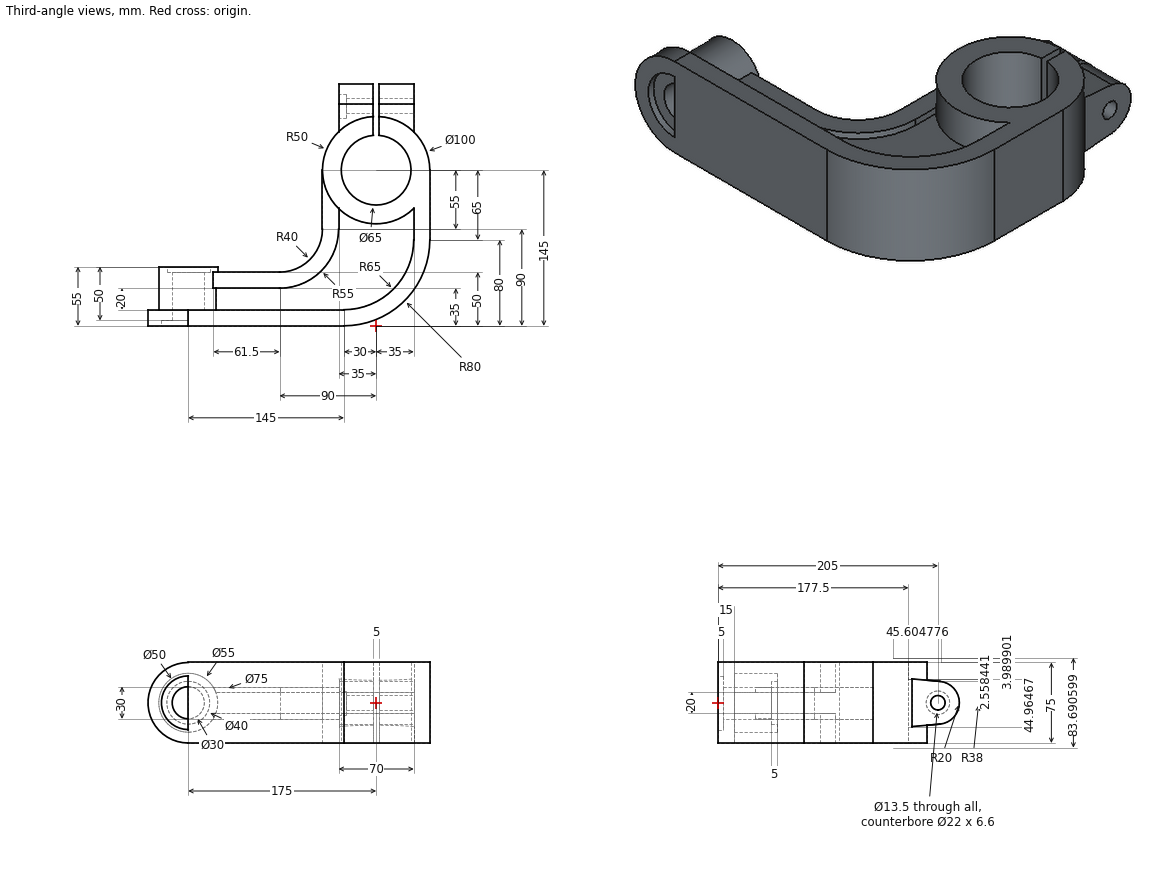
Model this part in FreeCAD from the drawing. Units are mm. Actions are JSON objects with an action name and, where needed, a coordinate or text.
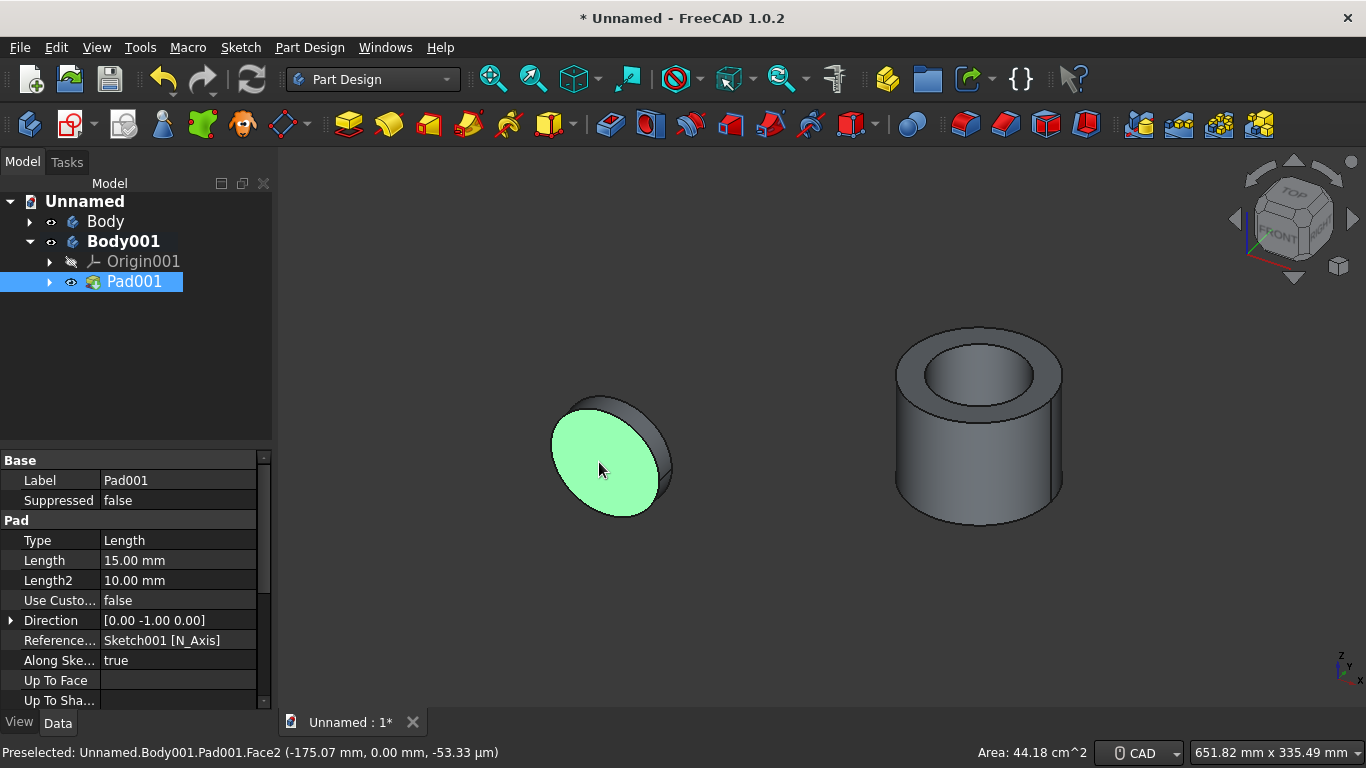
{"action": "left_click", "coordinate": [70, 124]}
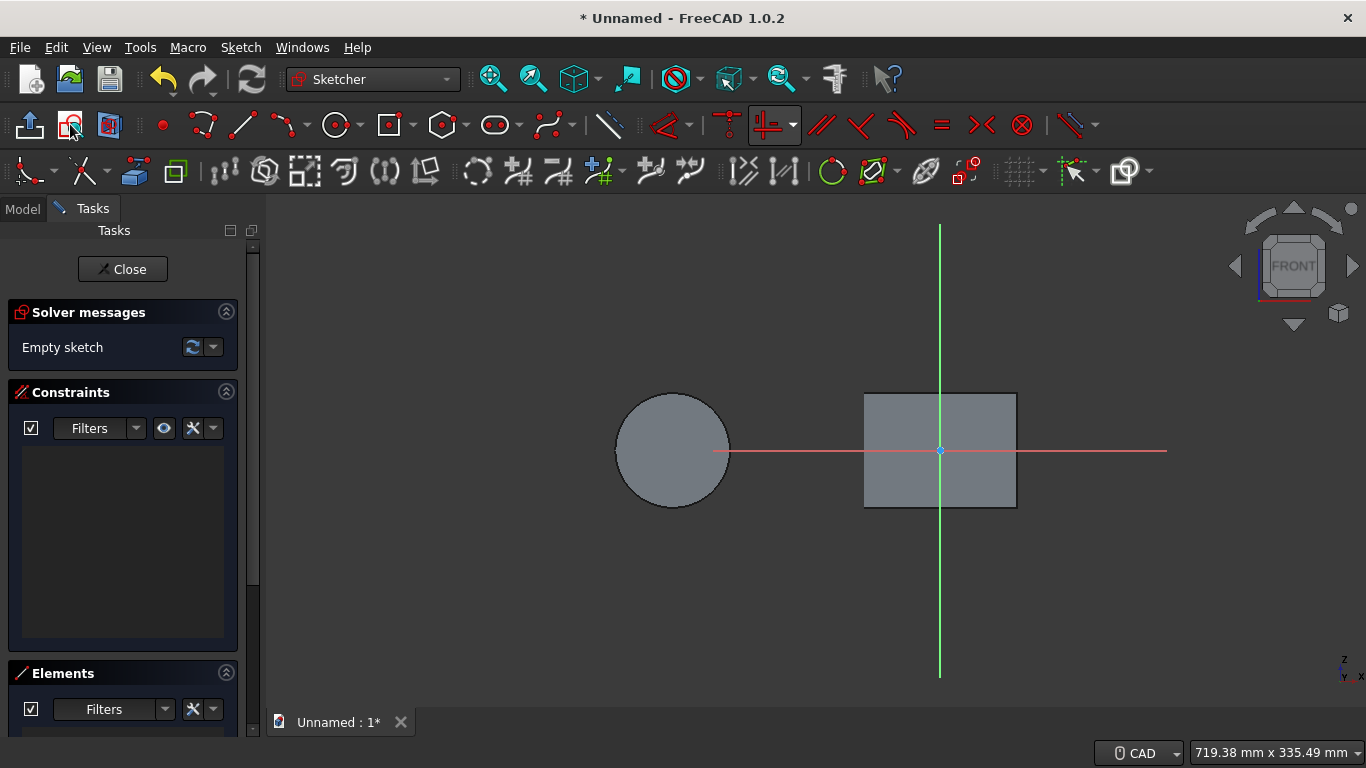
{"action": "scroll", "coordinate": [648, 450], "scroll_direction": "up", "scroll_amount": 7}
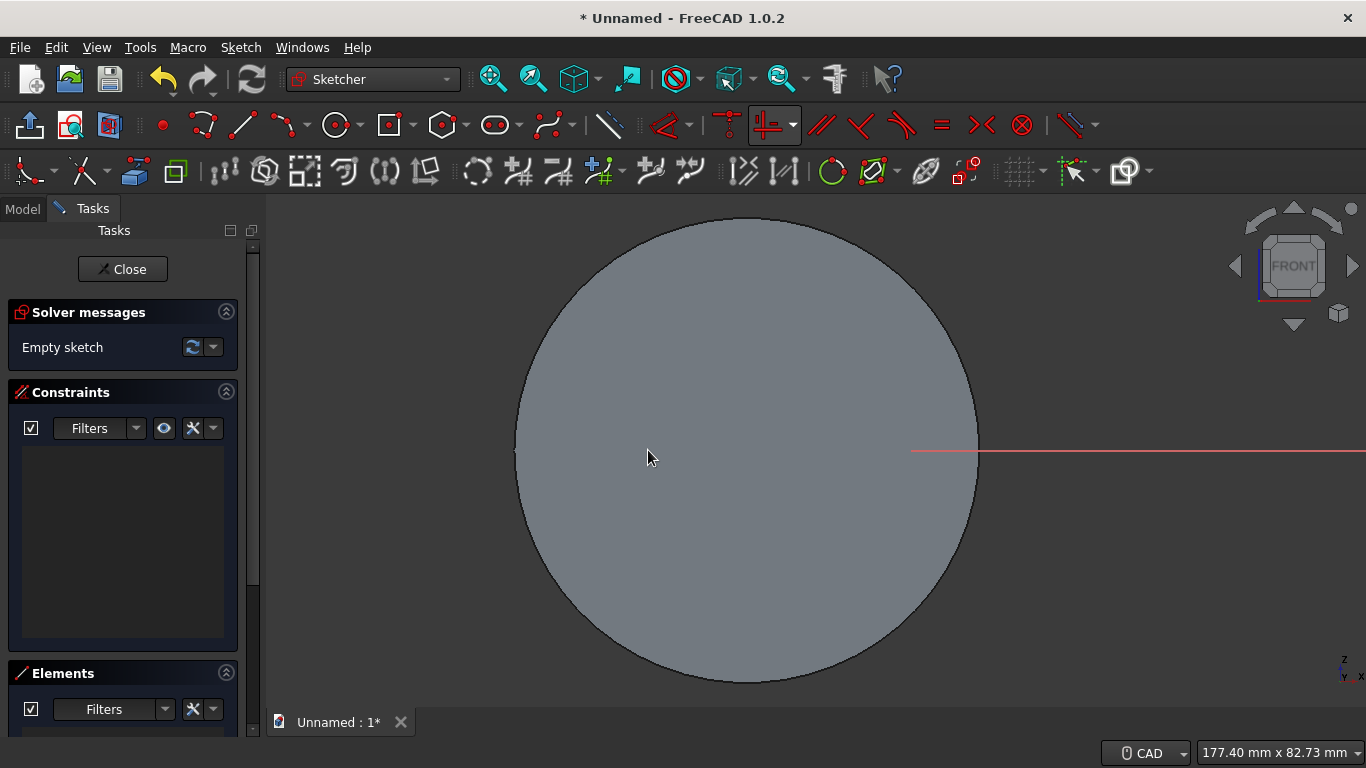
{"action": "key", "text": "g c"}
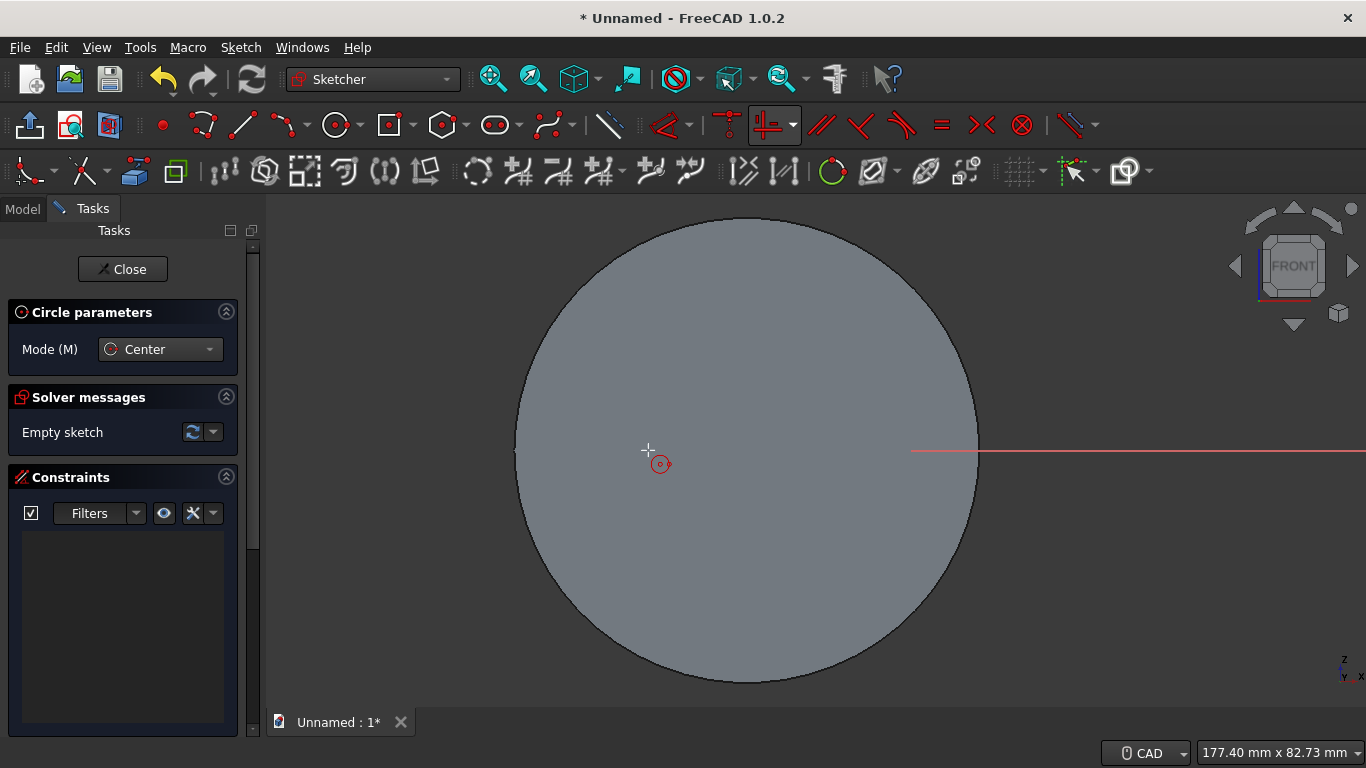
{"action": "left_click", "coordinate": [747, 450]}
{"action": "left_click", "coordinate": [867, 330]}
{"action": "key", "text": "Escape"}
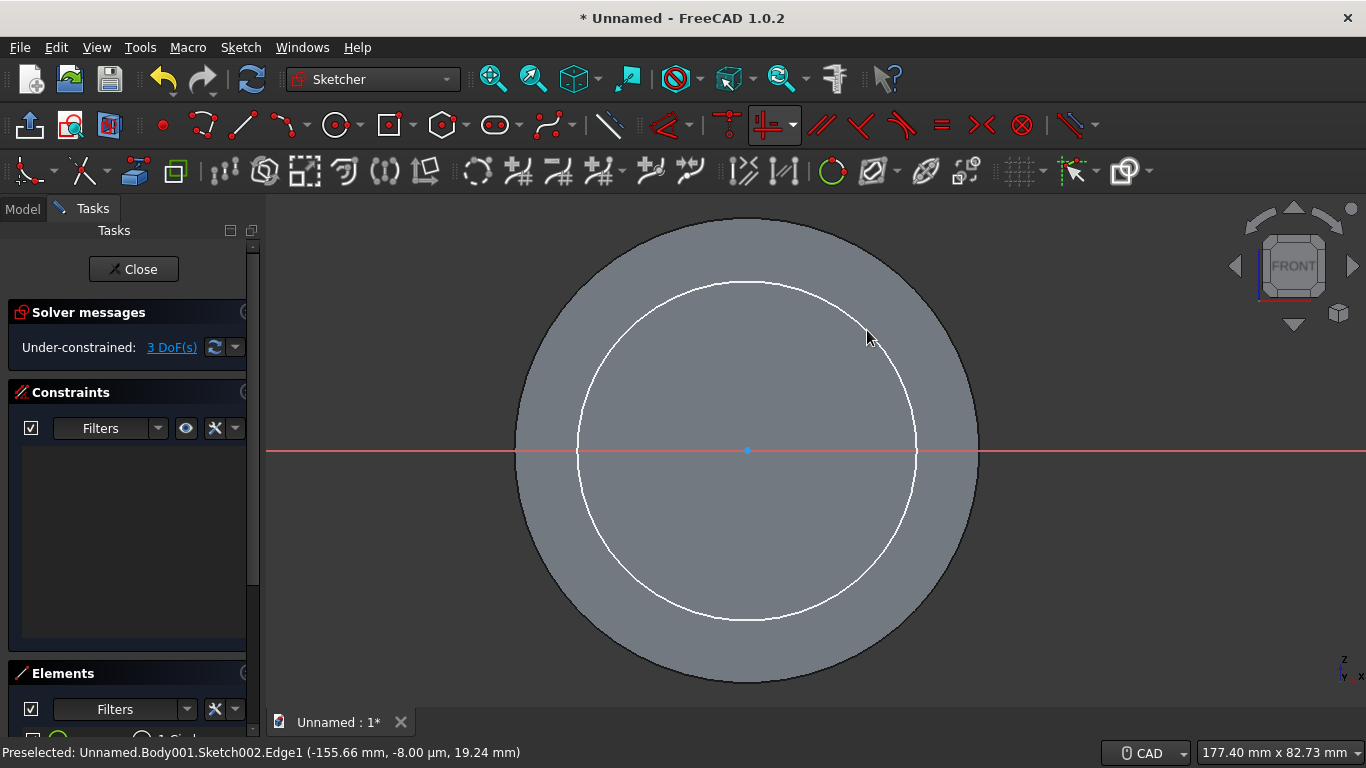
{"action": "left_click", "coordinate": [747, 451]}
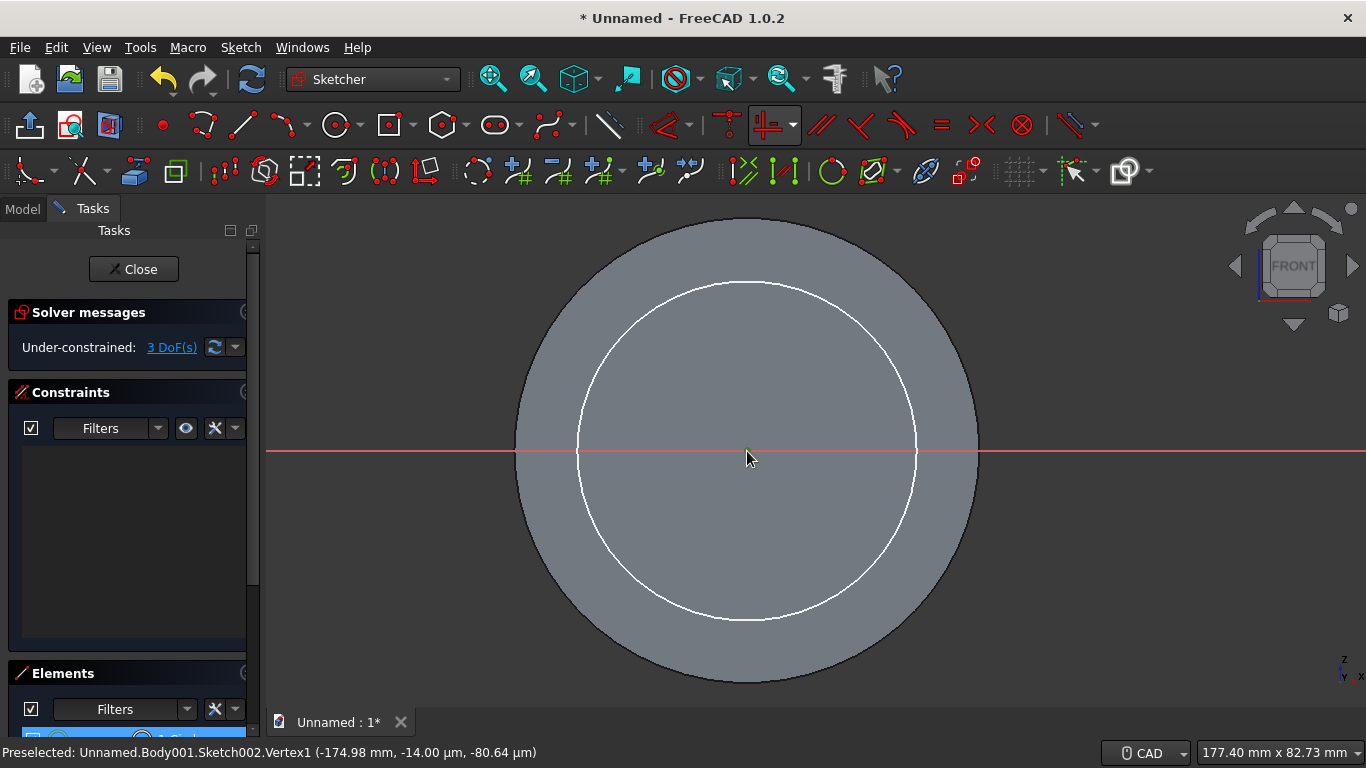
{"action": "left_click", "coordinate": [359, 450]}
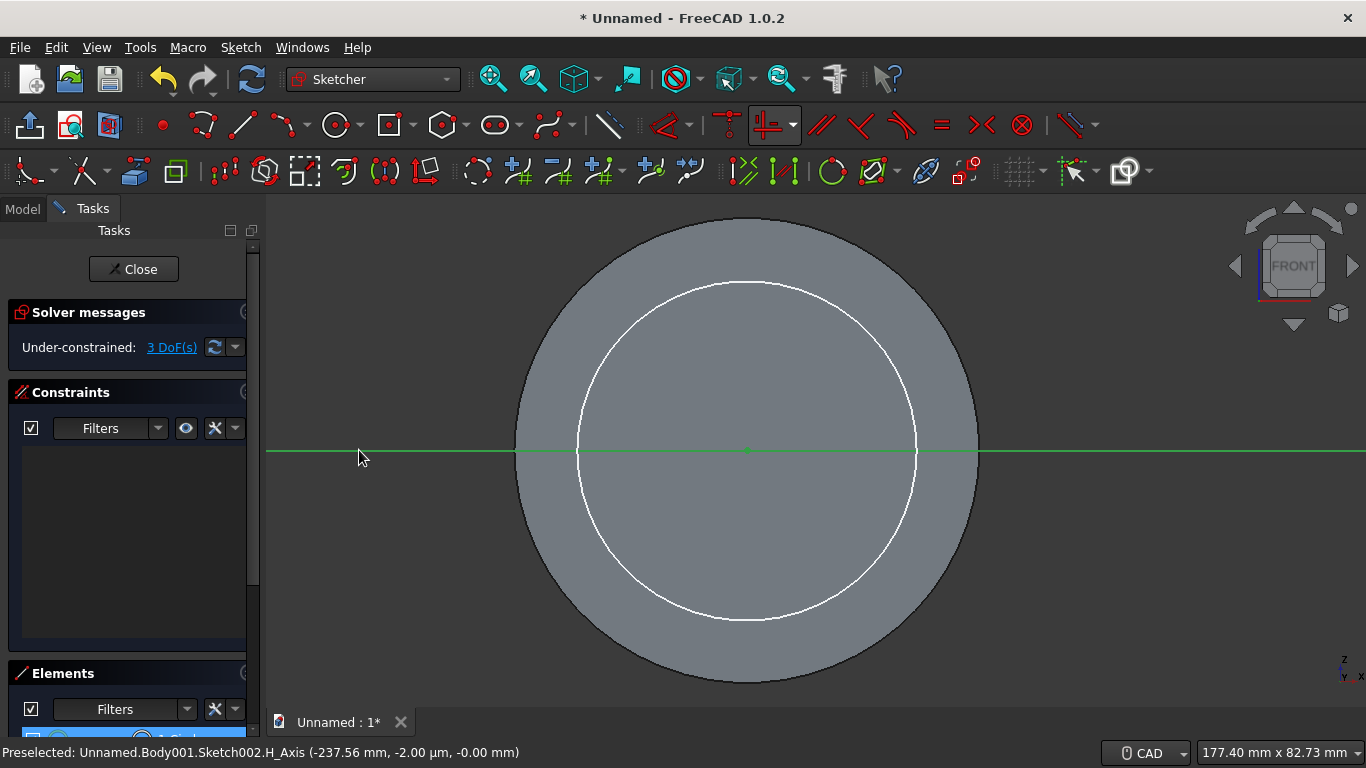
{"action": "key", "text": "c"}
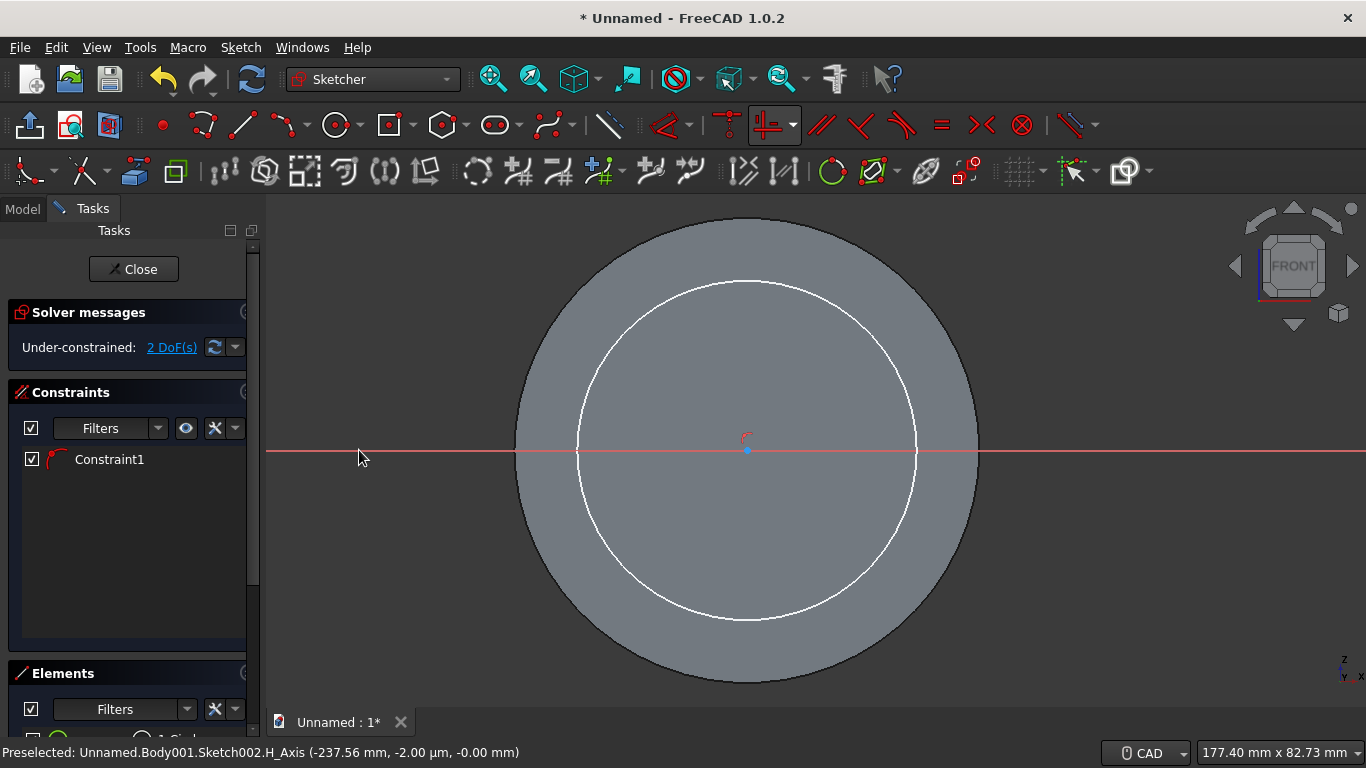
{"action": "key", "text": "d"}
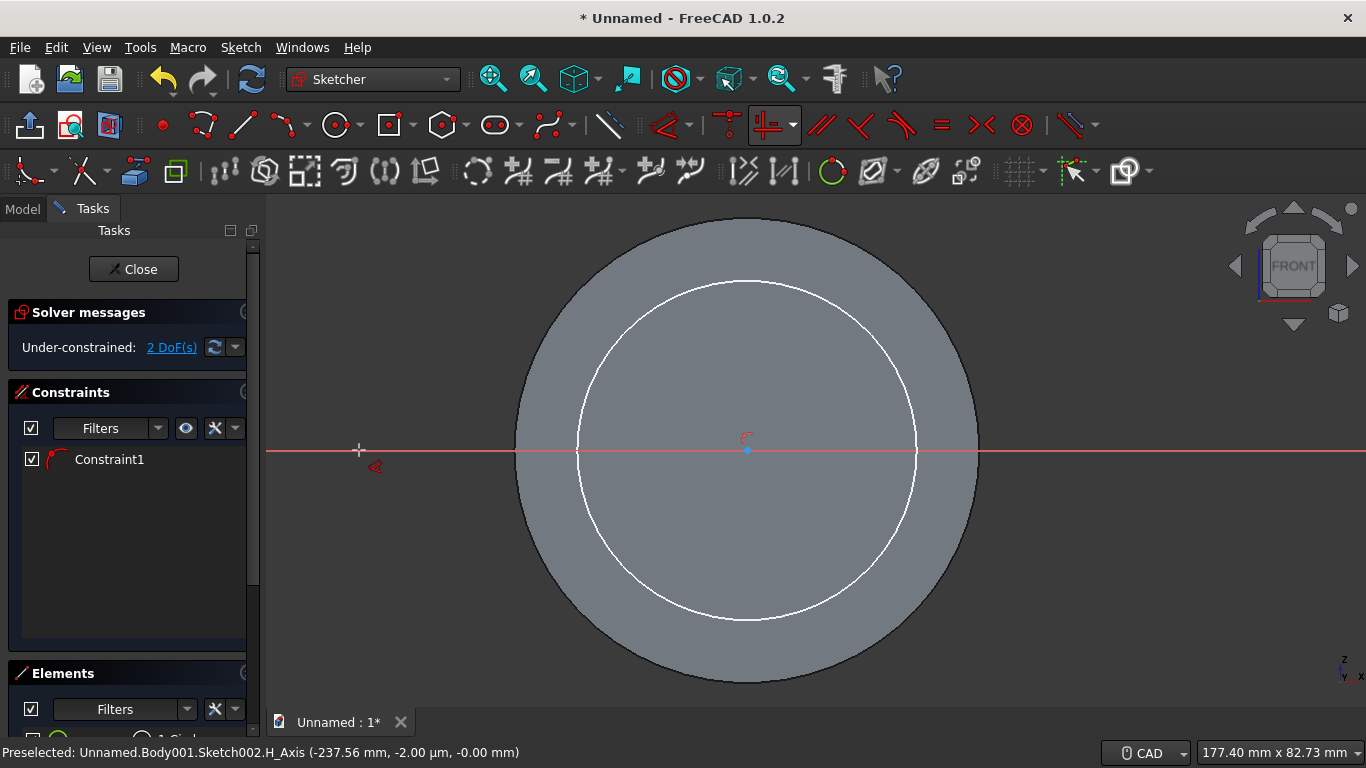
{"action": "left_click", "coordinate": [867, 330]}
{"action": "left_click", "coordinate": [890, 307]}